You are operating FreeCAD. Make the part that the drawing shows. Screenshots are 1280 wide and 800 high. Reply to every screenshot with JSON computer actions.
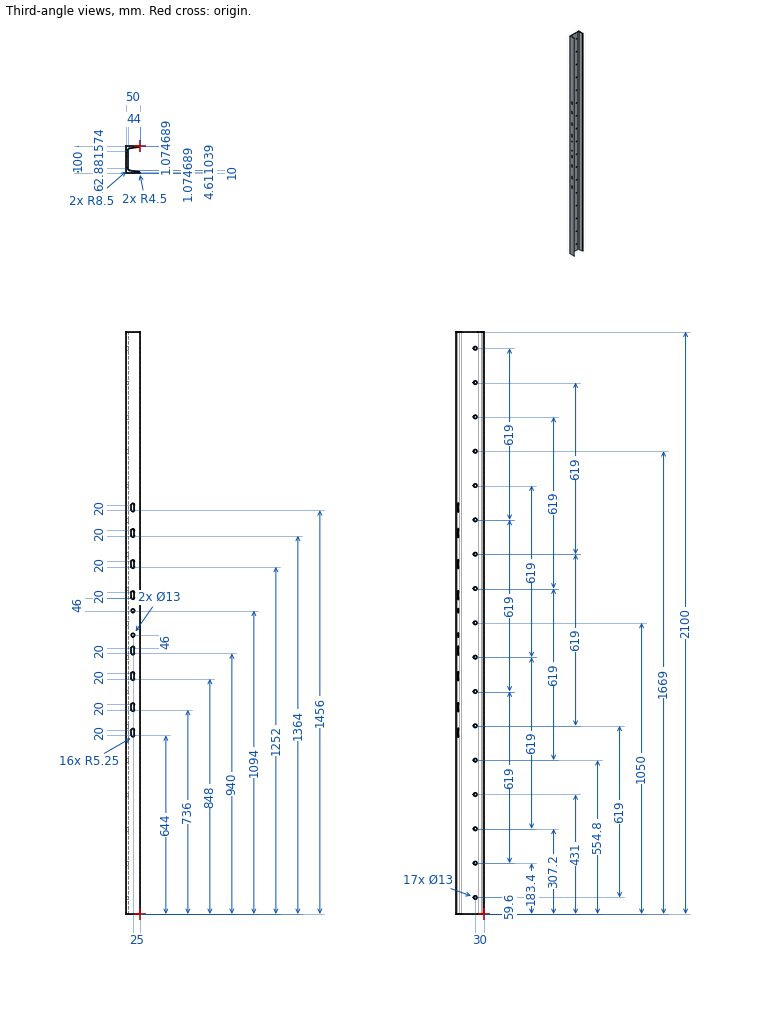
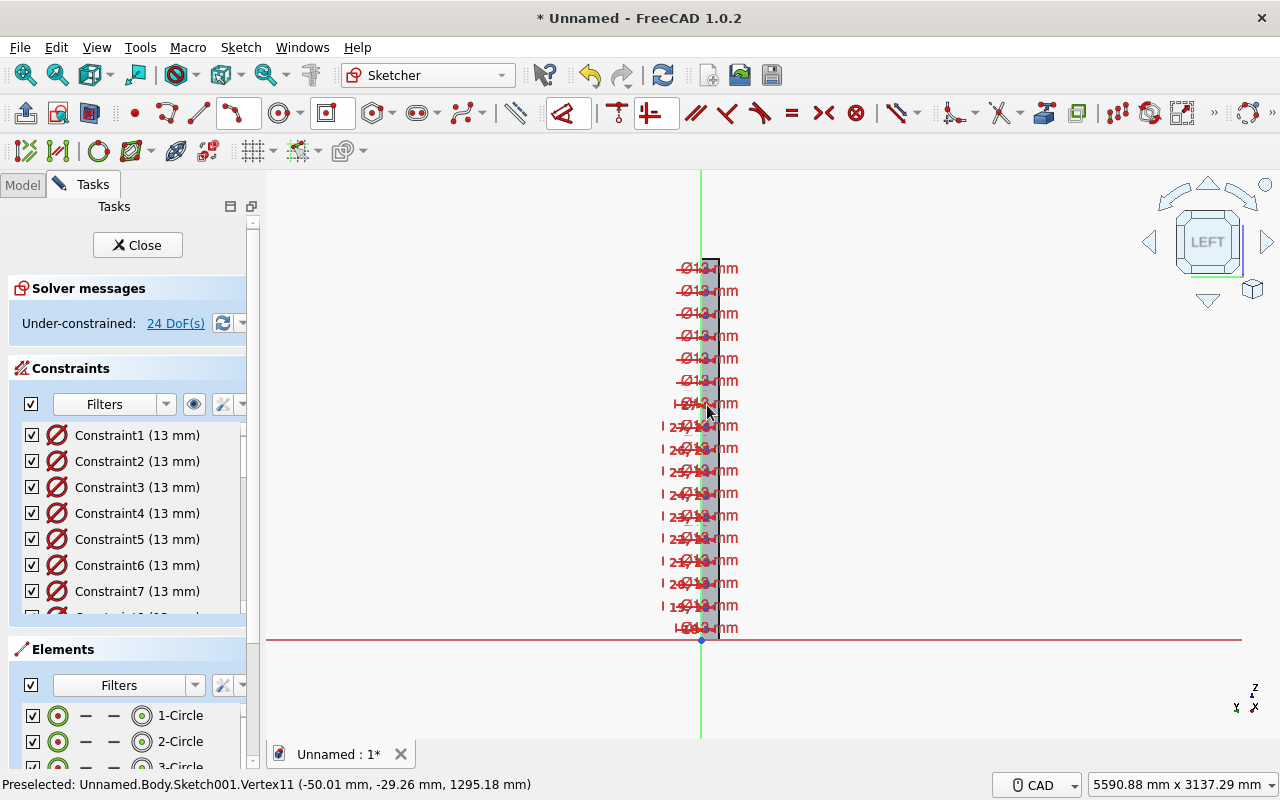
{"action": "left_click", "coordinate": [707, 383]}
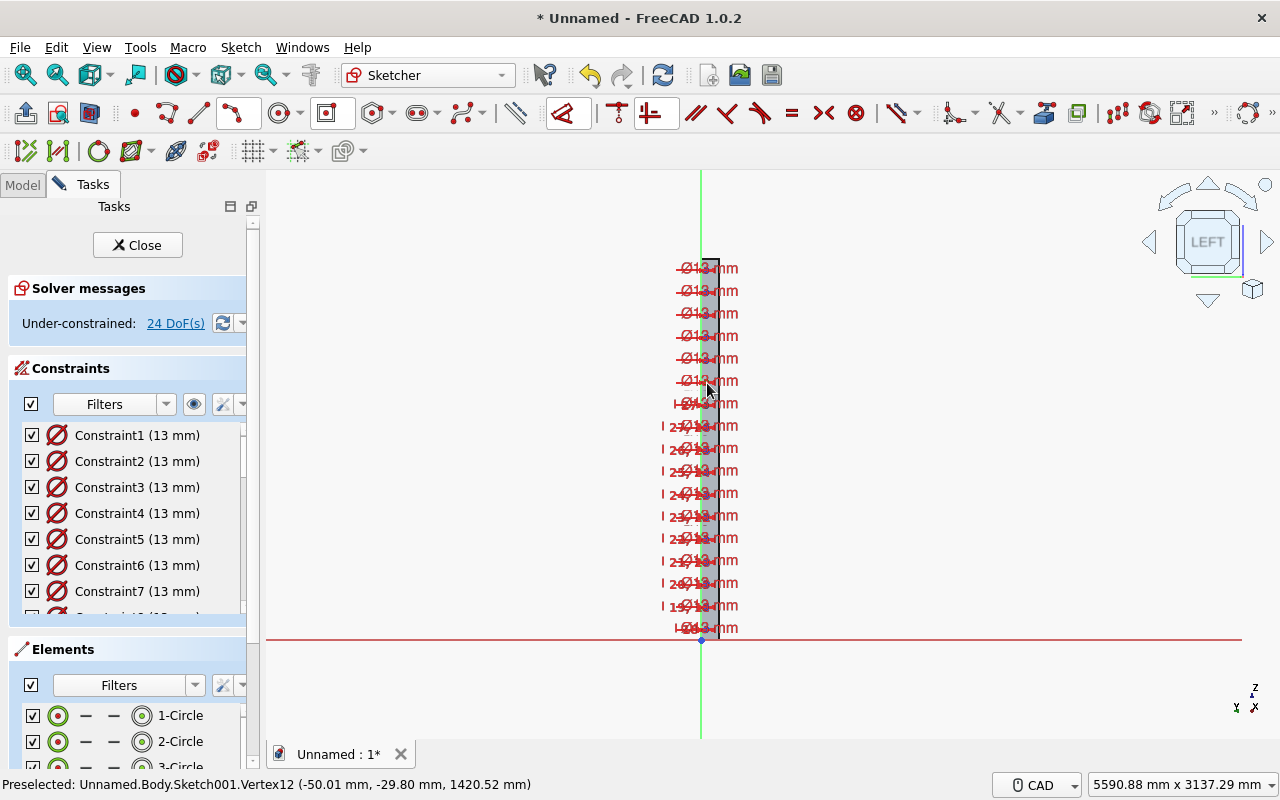
{"action": "key", "text": "v"}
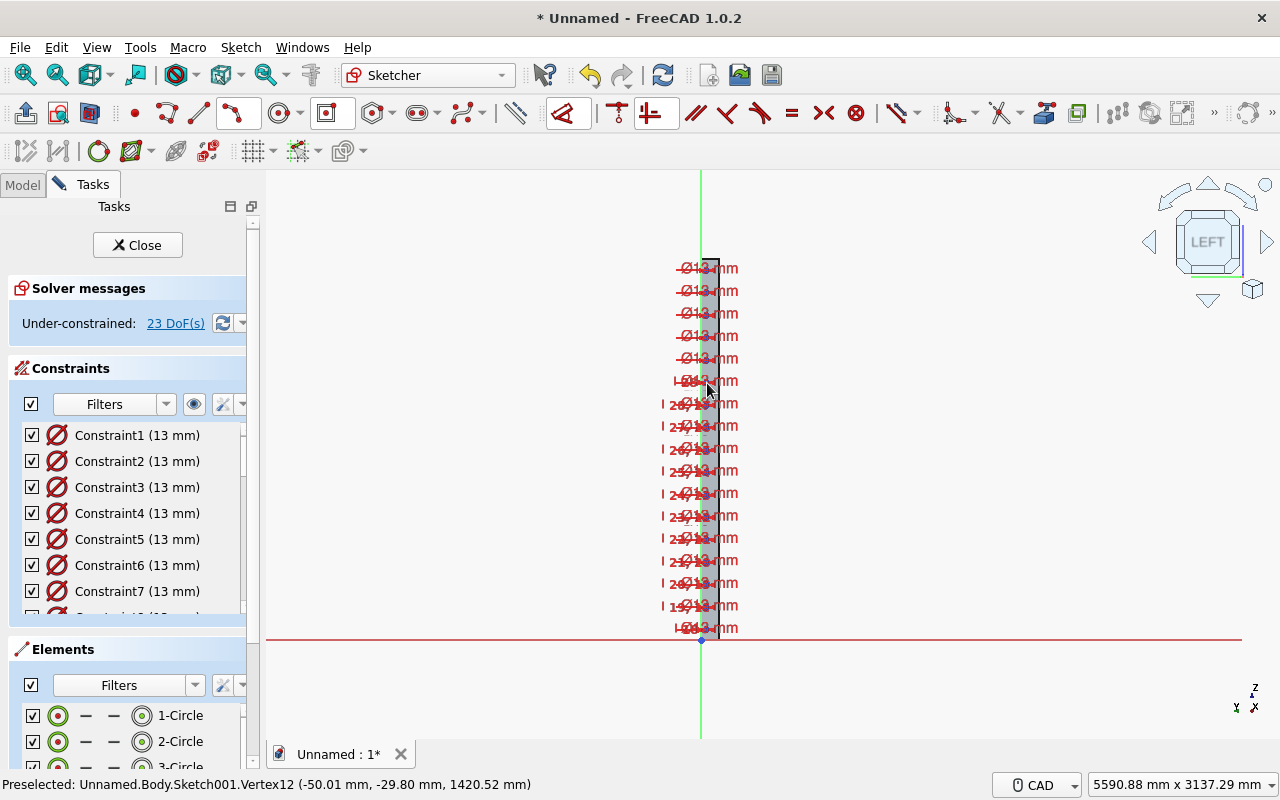
{"action": "left_click", "coordinate": [707, 383]}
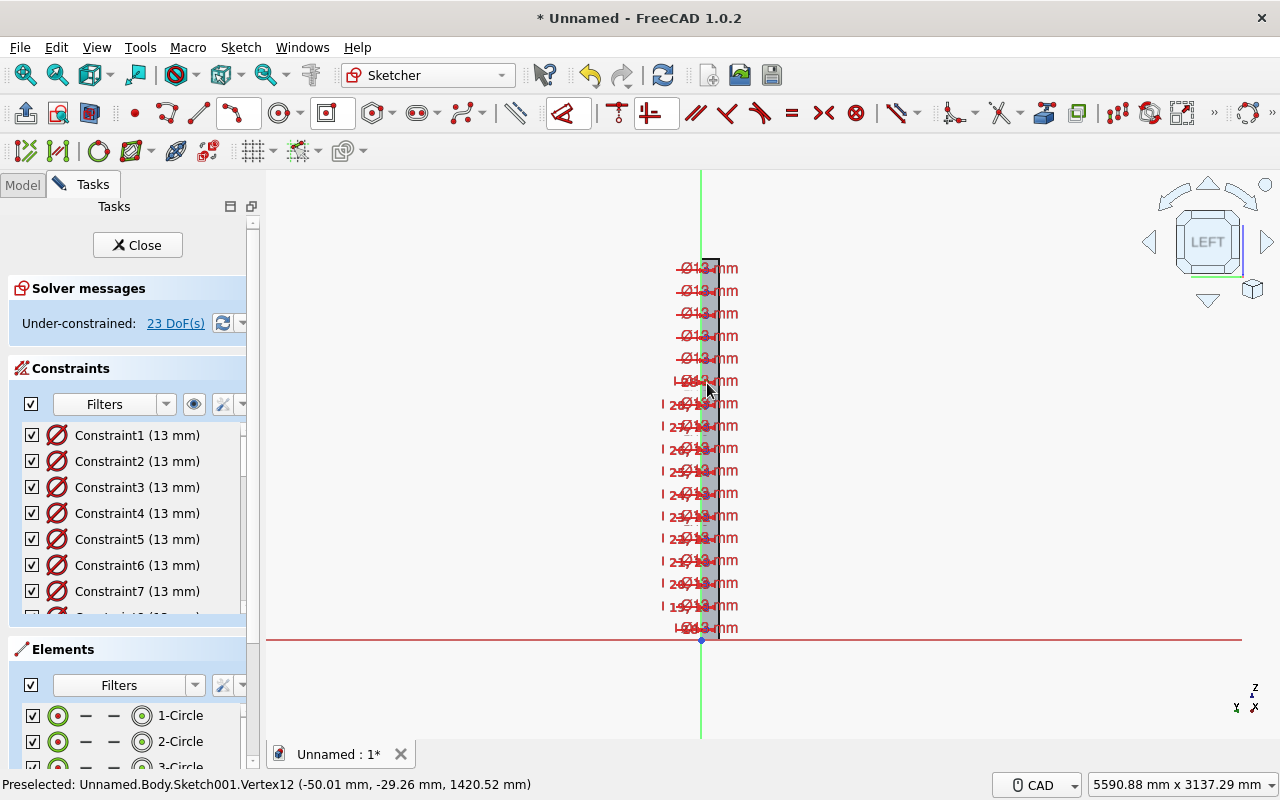
{"action": "left_click", "coordinate": [707, 360]}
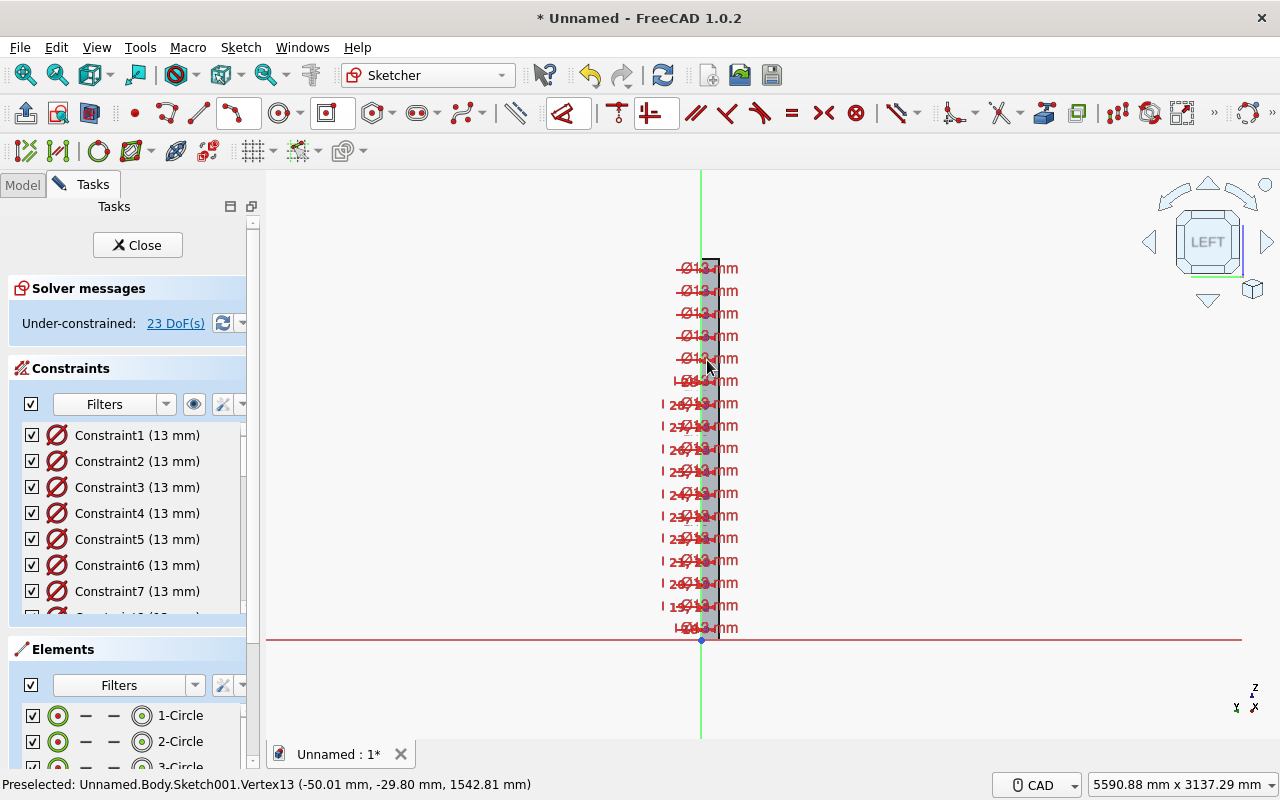
{"action": "key", "text": "v"}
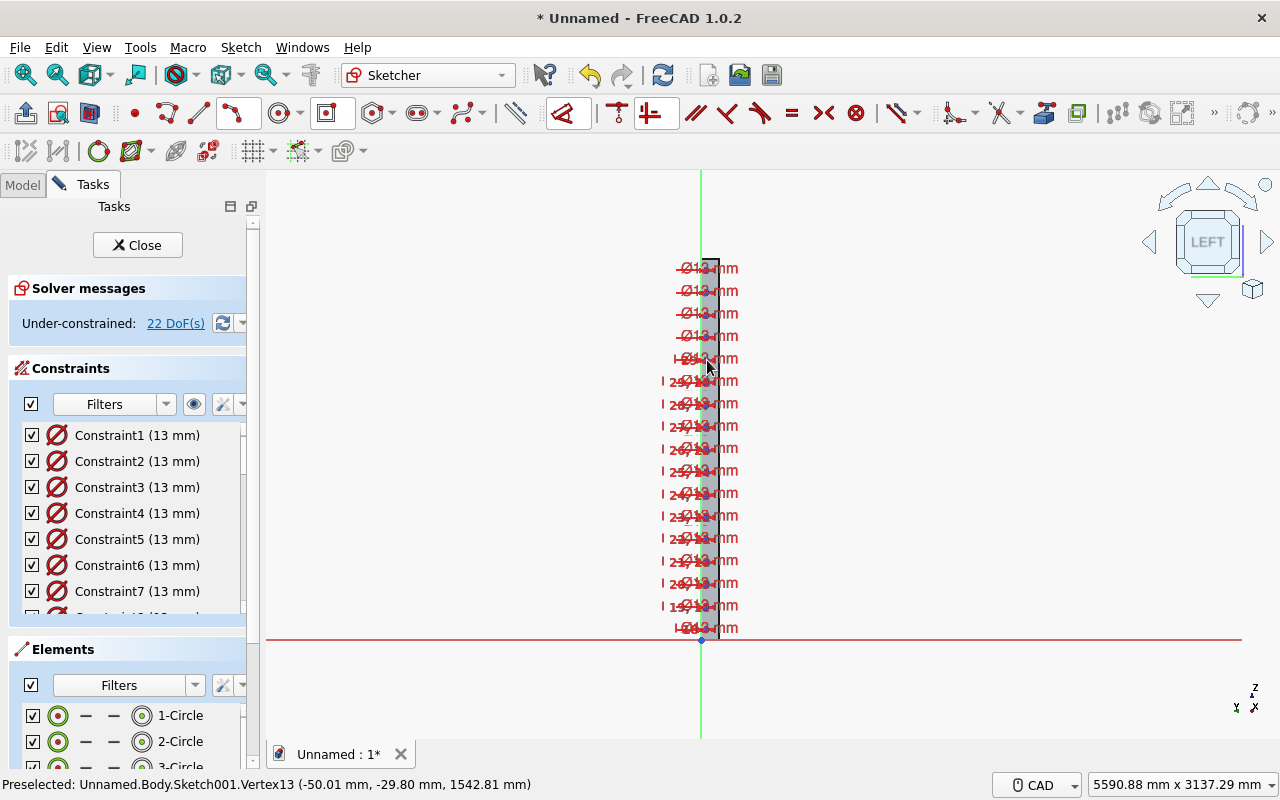
{"action": "left_click", "coordinate": [707, 360]}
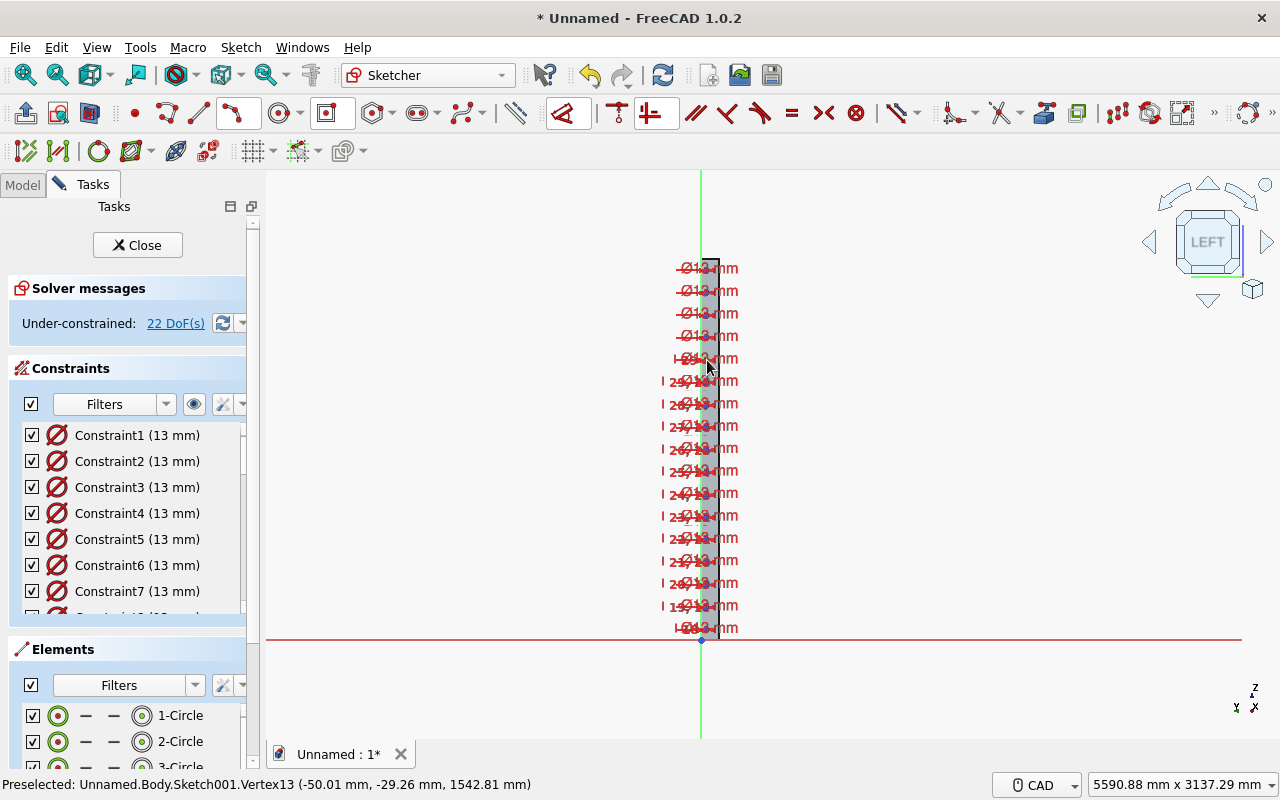
{"action": "left_click", "coordinate": [707, 338]}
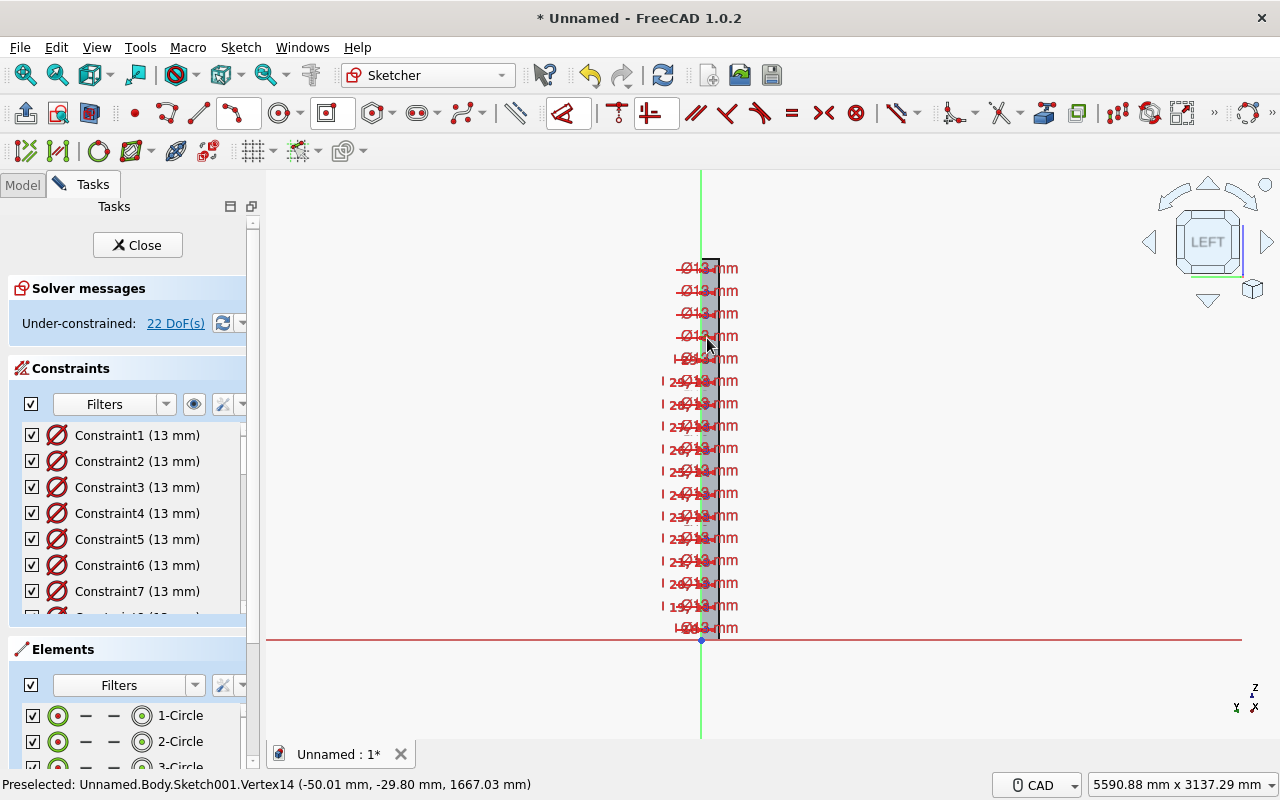
{"action": "key", "text": "v"}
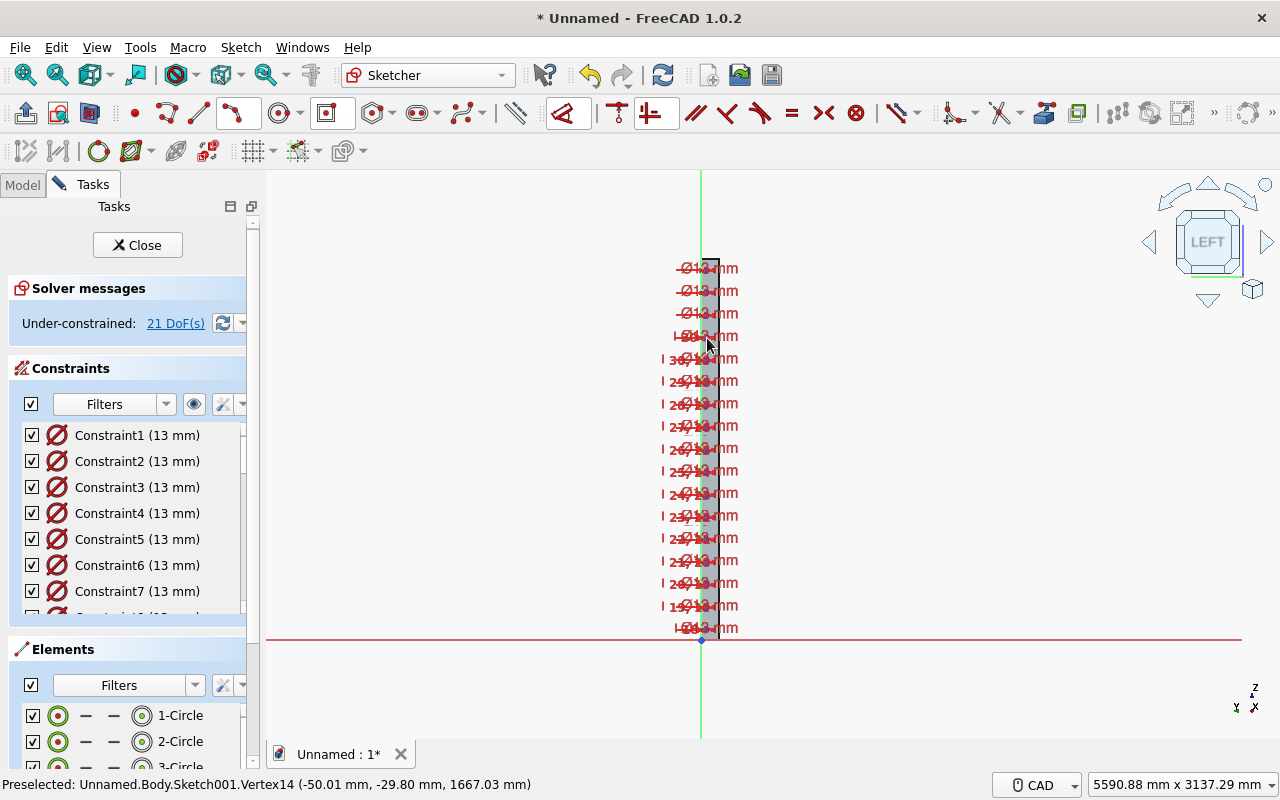
{"action": "left_click", "coordinate": [707, 338]}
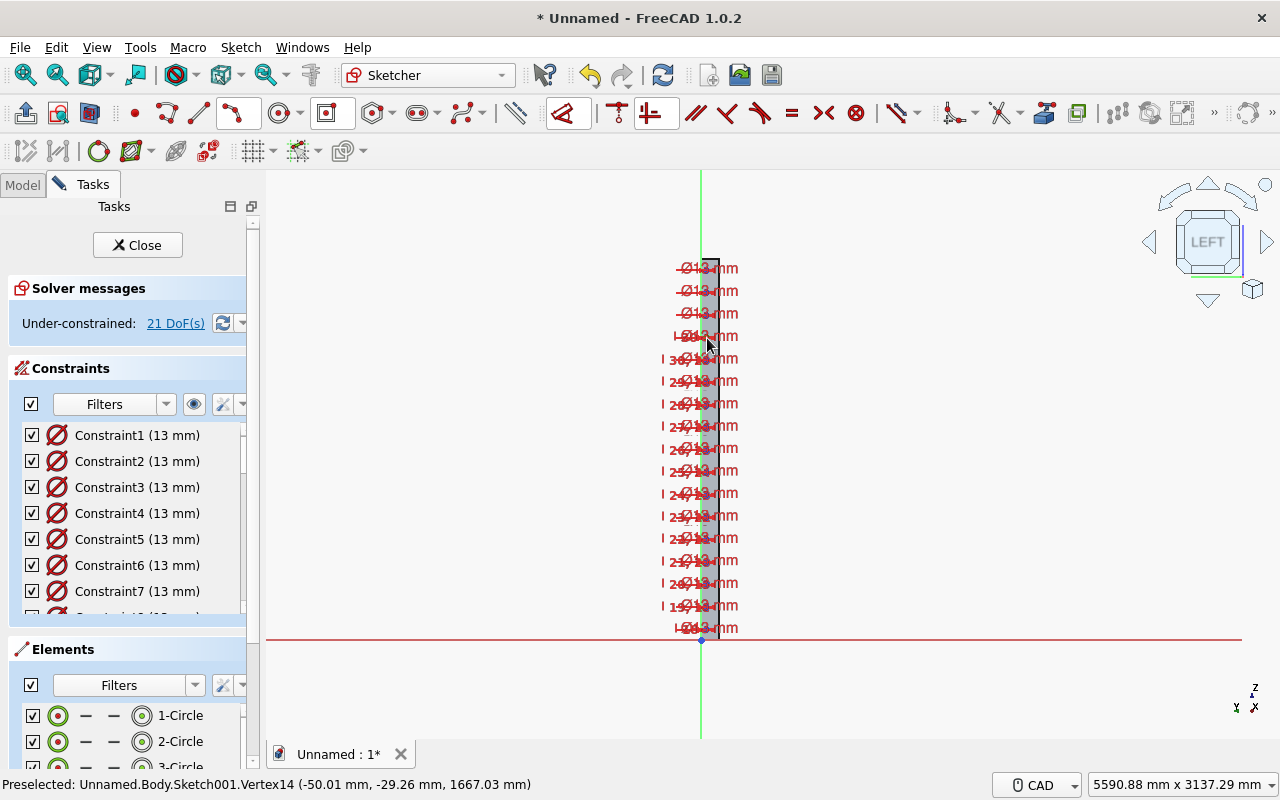
{"action": "left_click", "coordinate": [707, 315]}